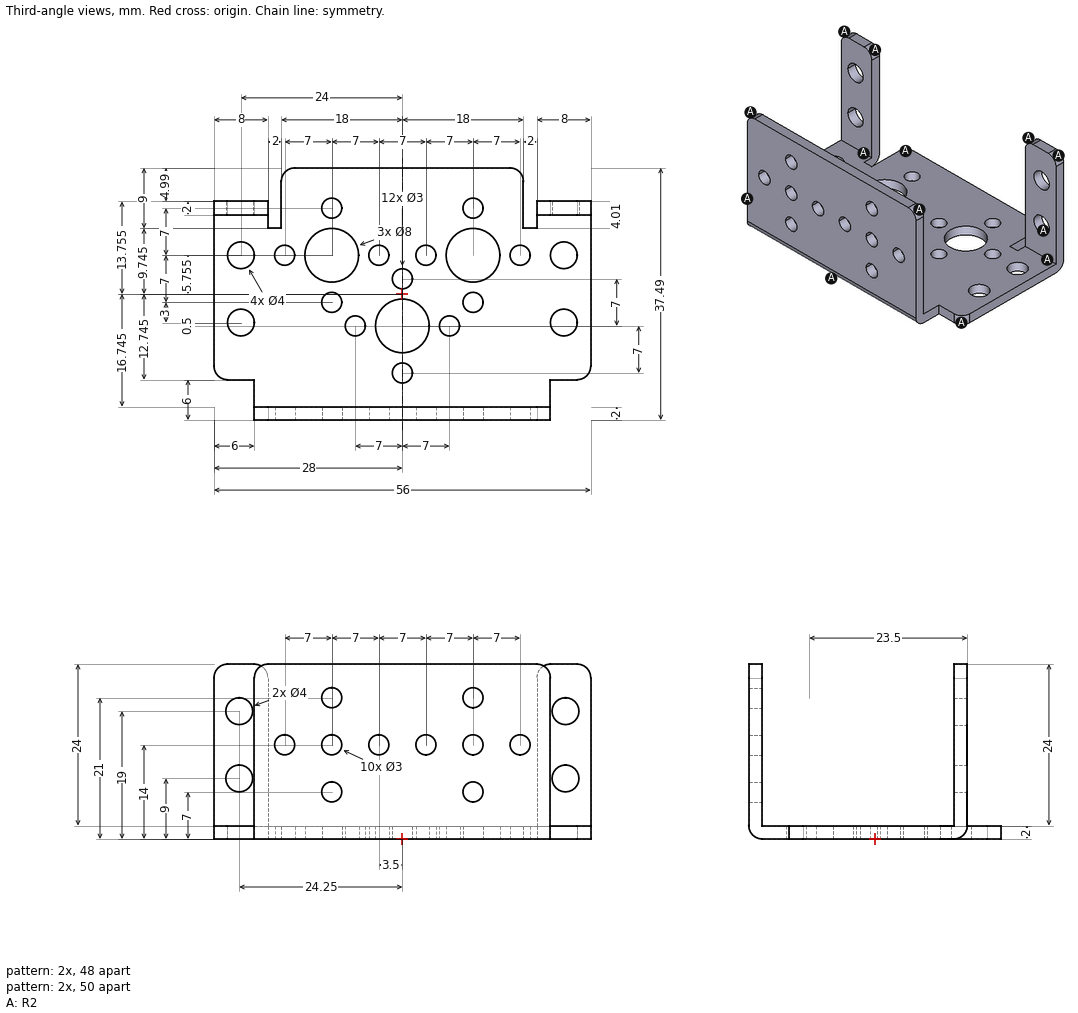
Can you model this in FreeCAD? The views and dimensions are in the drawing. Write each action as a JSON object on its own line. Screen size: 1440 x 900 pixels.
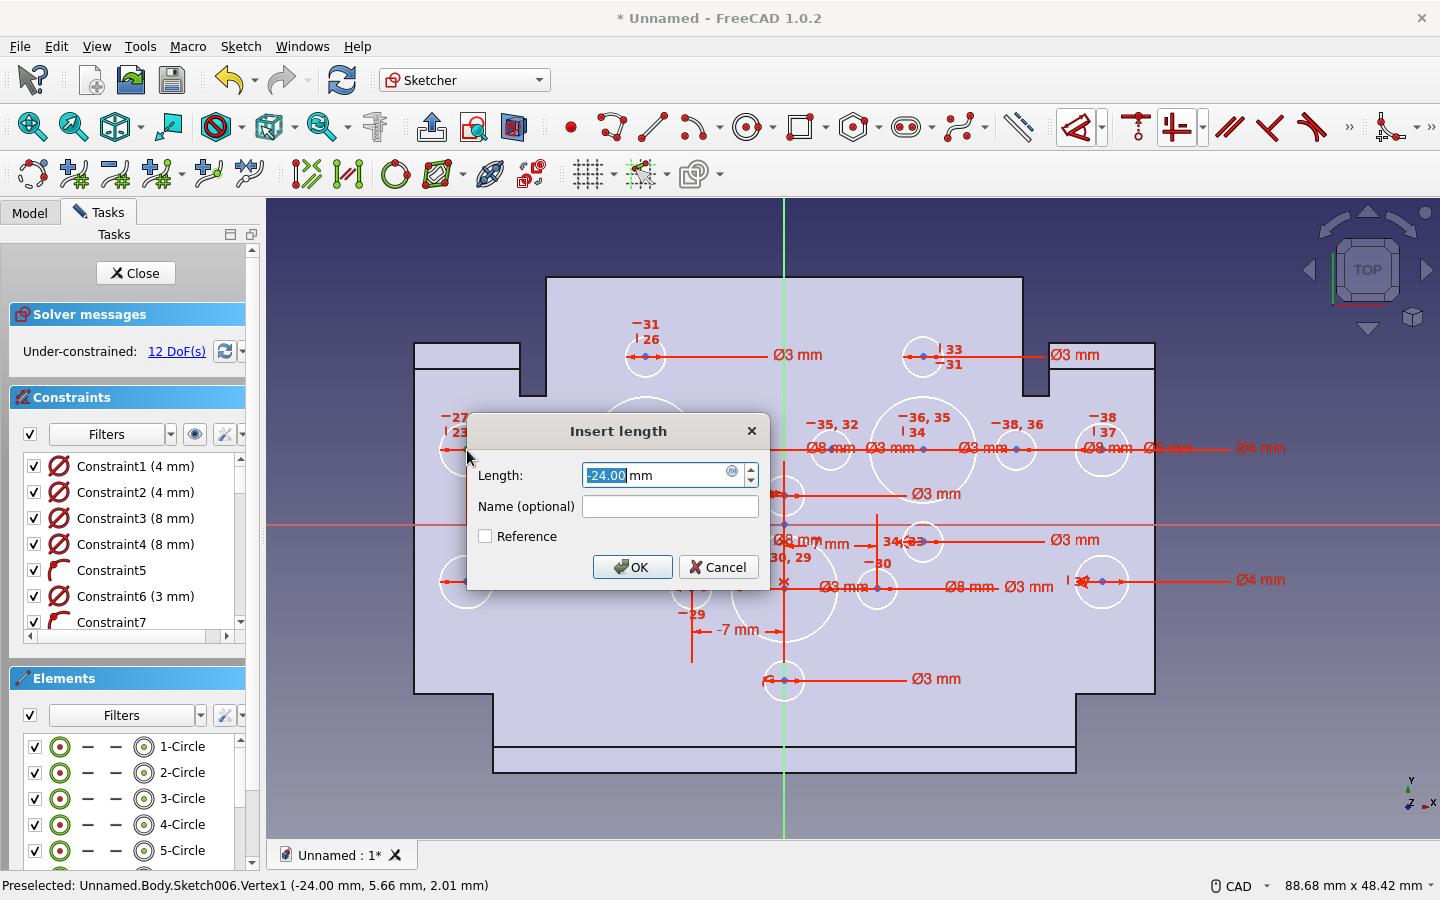
{"action": "type", "text": "-24"}
{"action": "key", "text": "Return"}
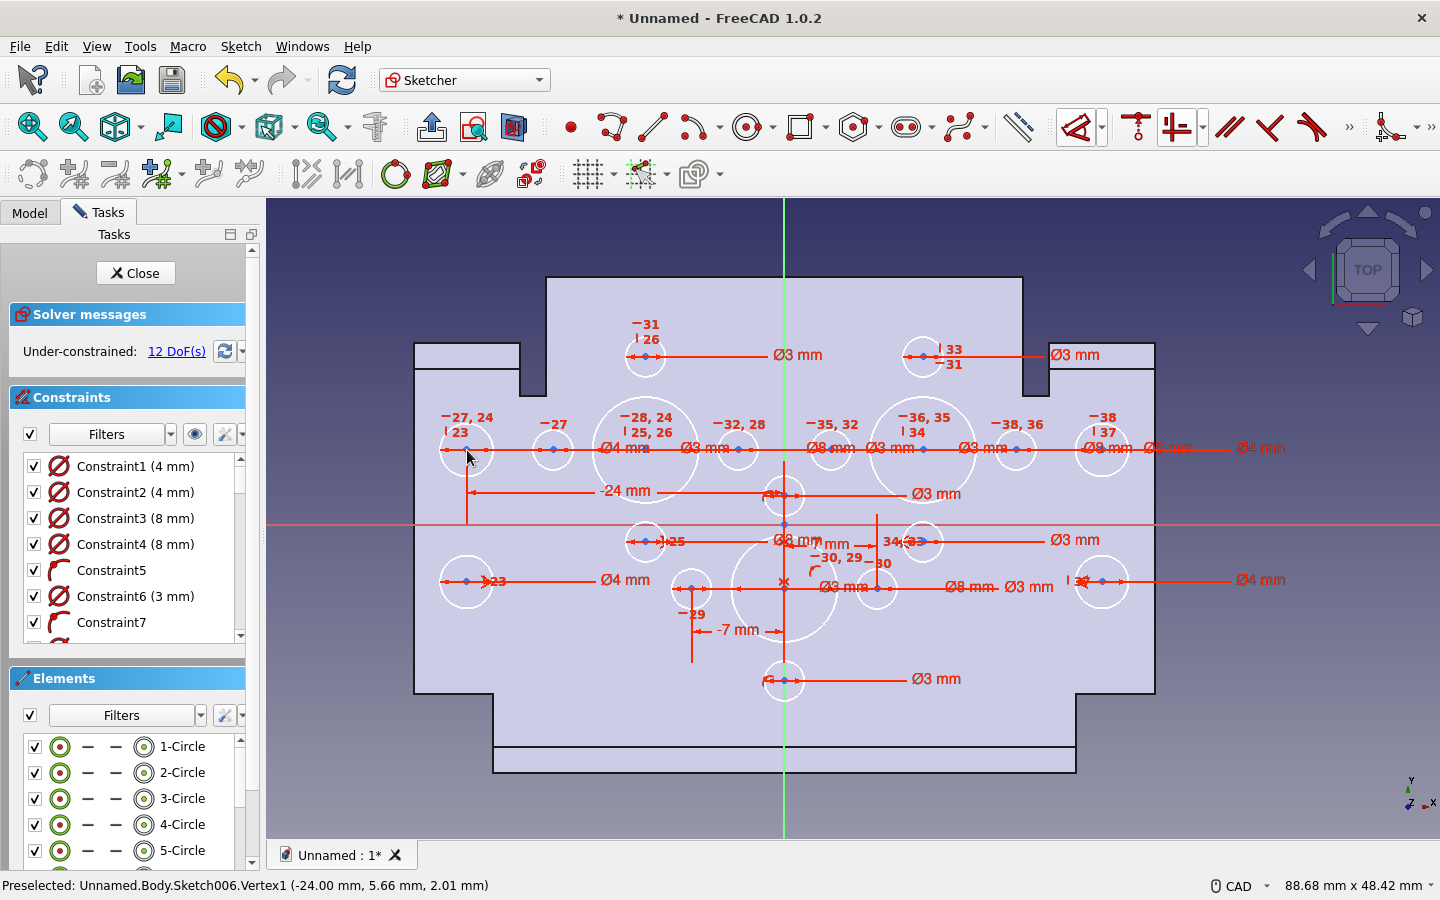
{"action": "left_click", "coordinate": [784, 589]}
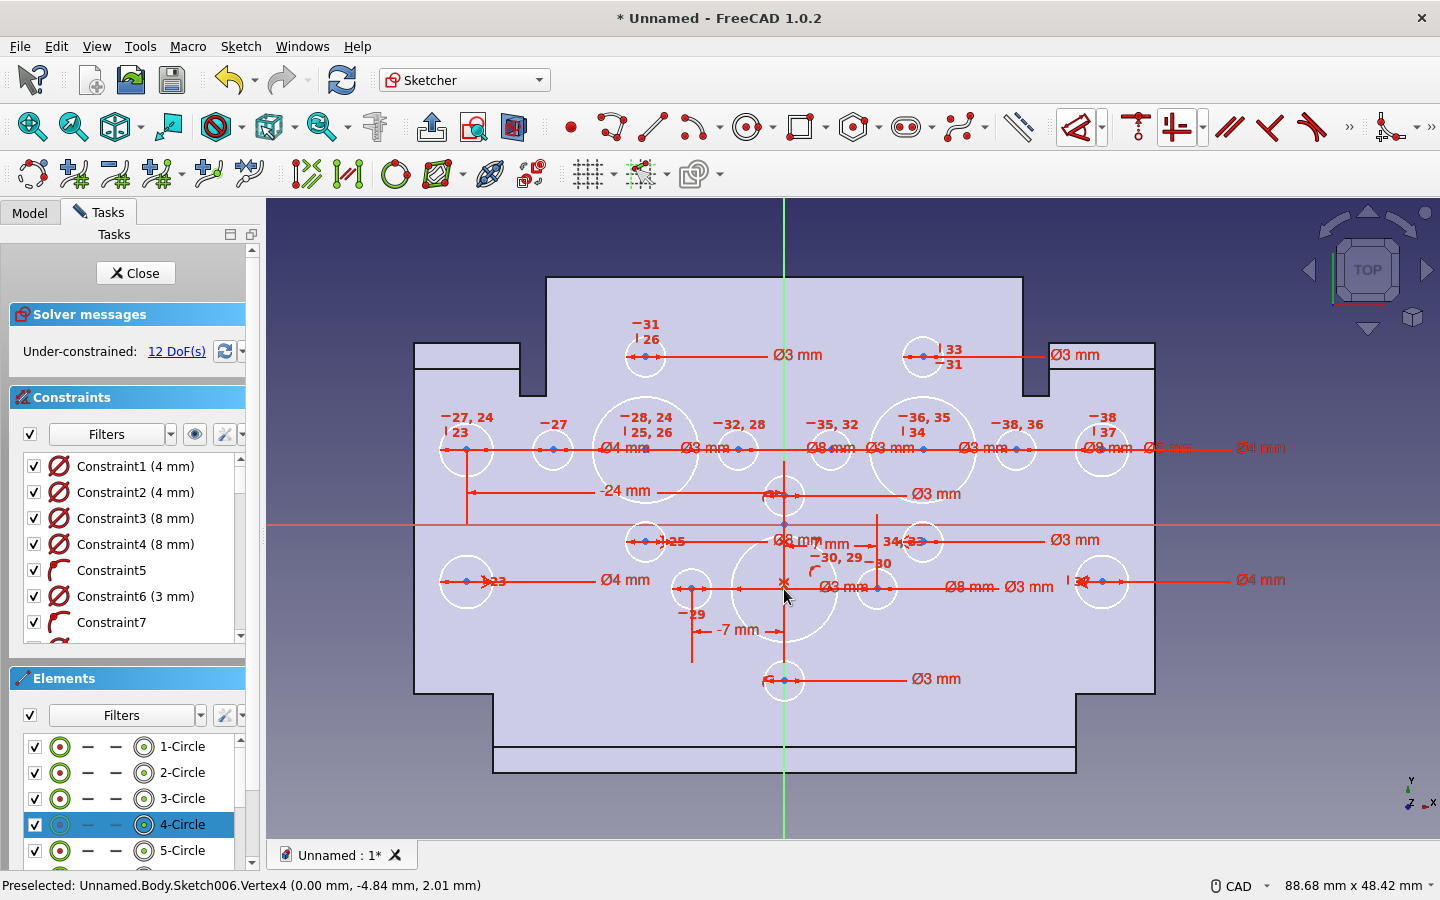
{"action": "left_click", "coordinate": [784, 496]}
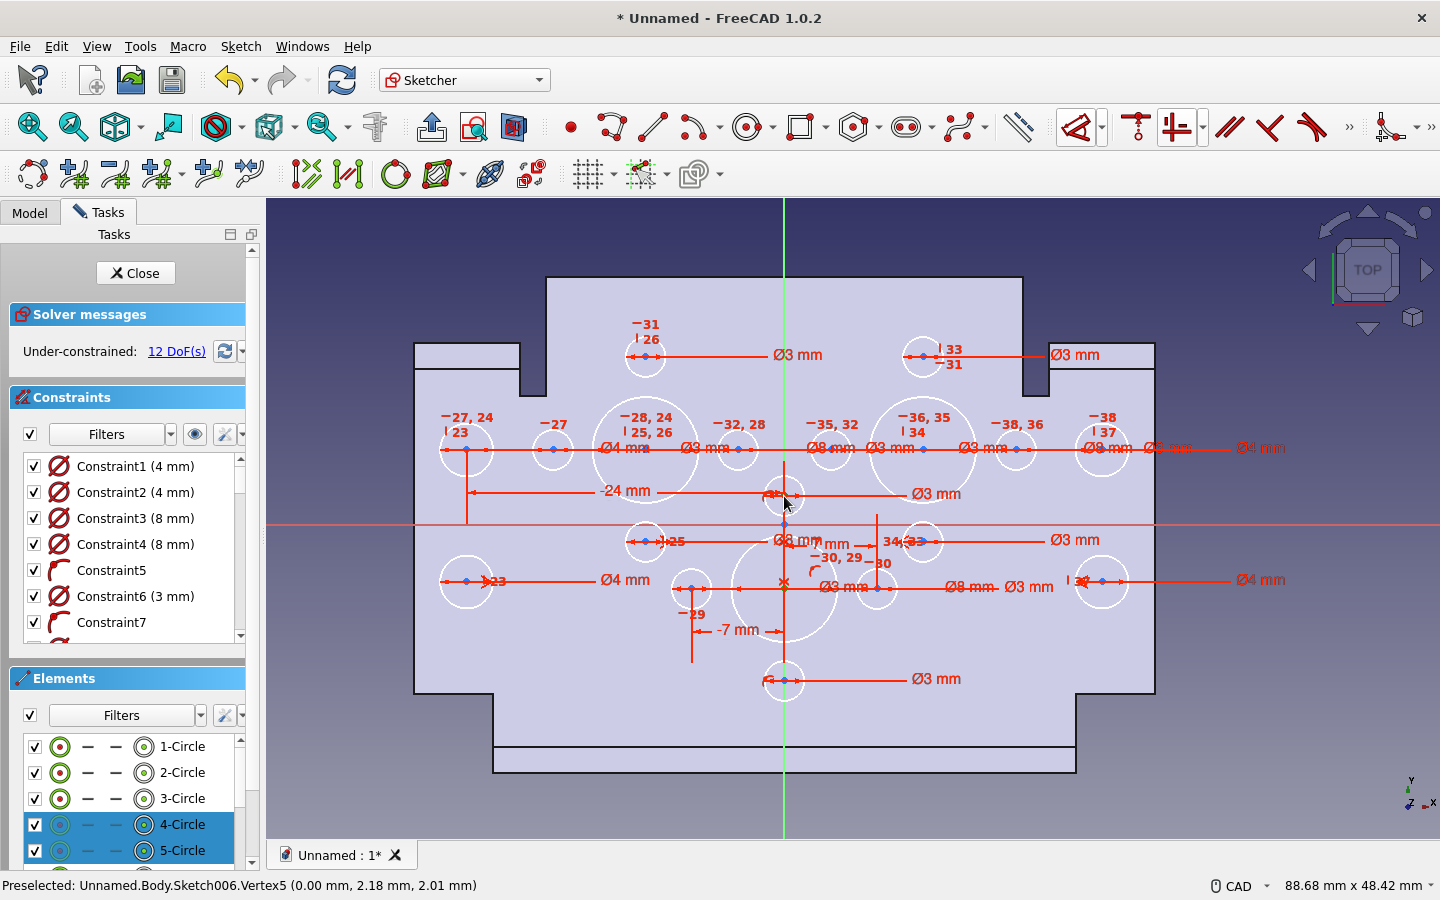
{"action": "key", "text": "i"}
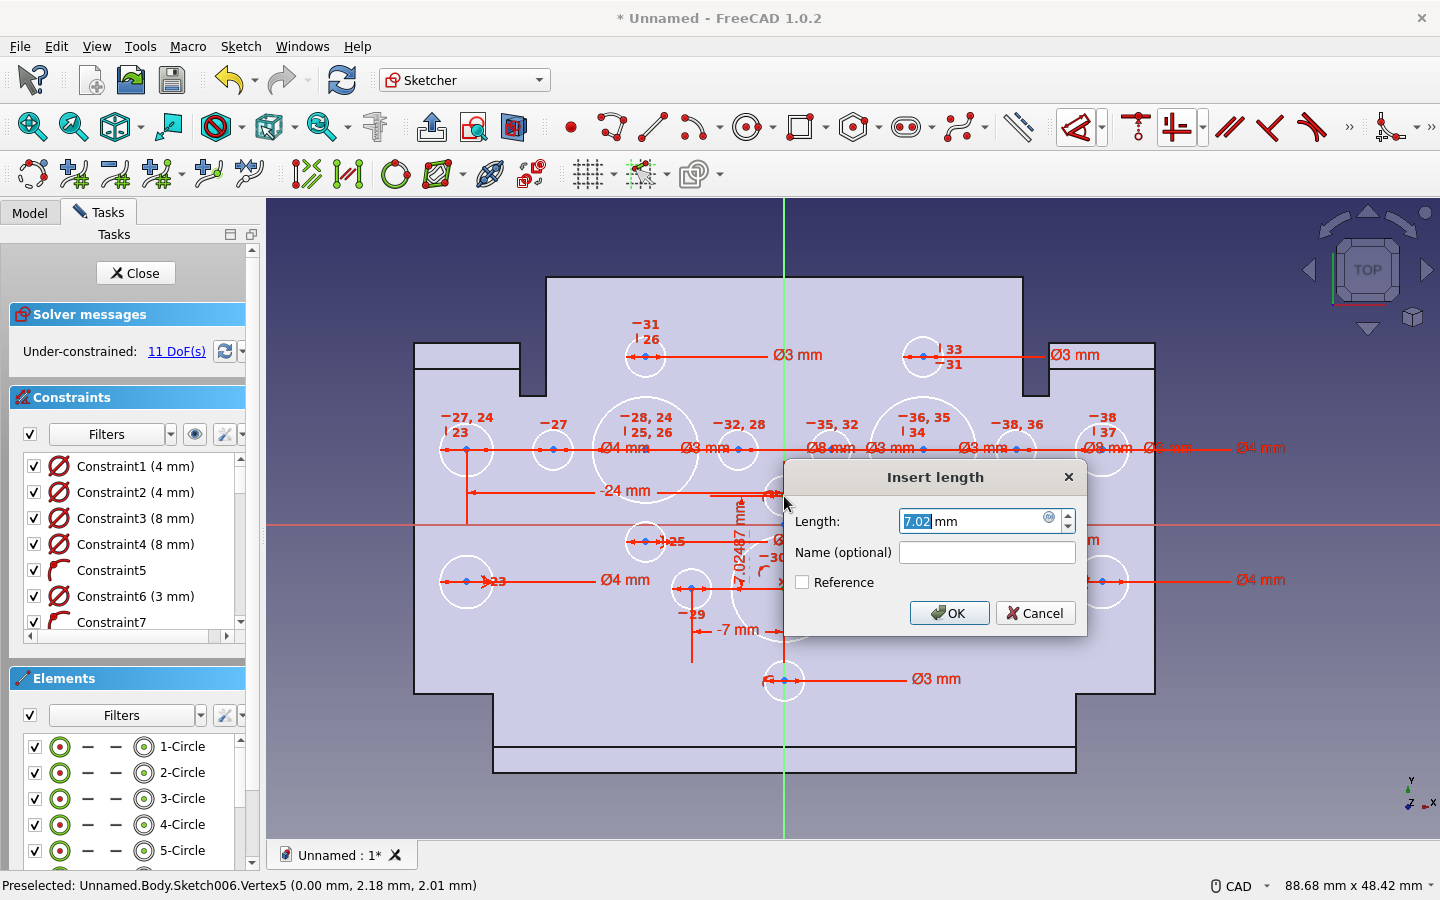
{"action": "type", "text": "7"}
{"action": "key", "text": "Return"}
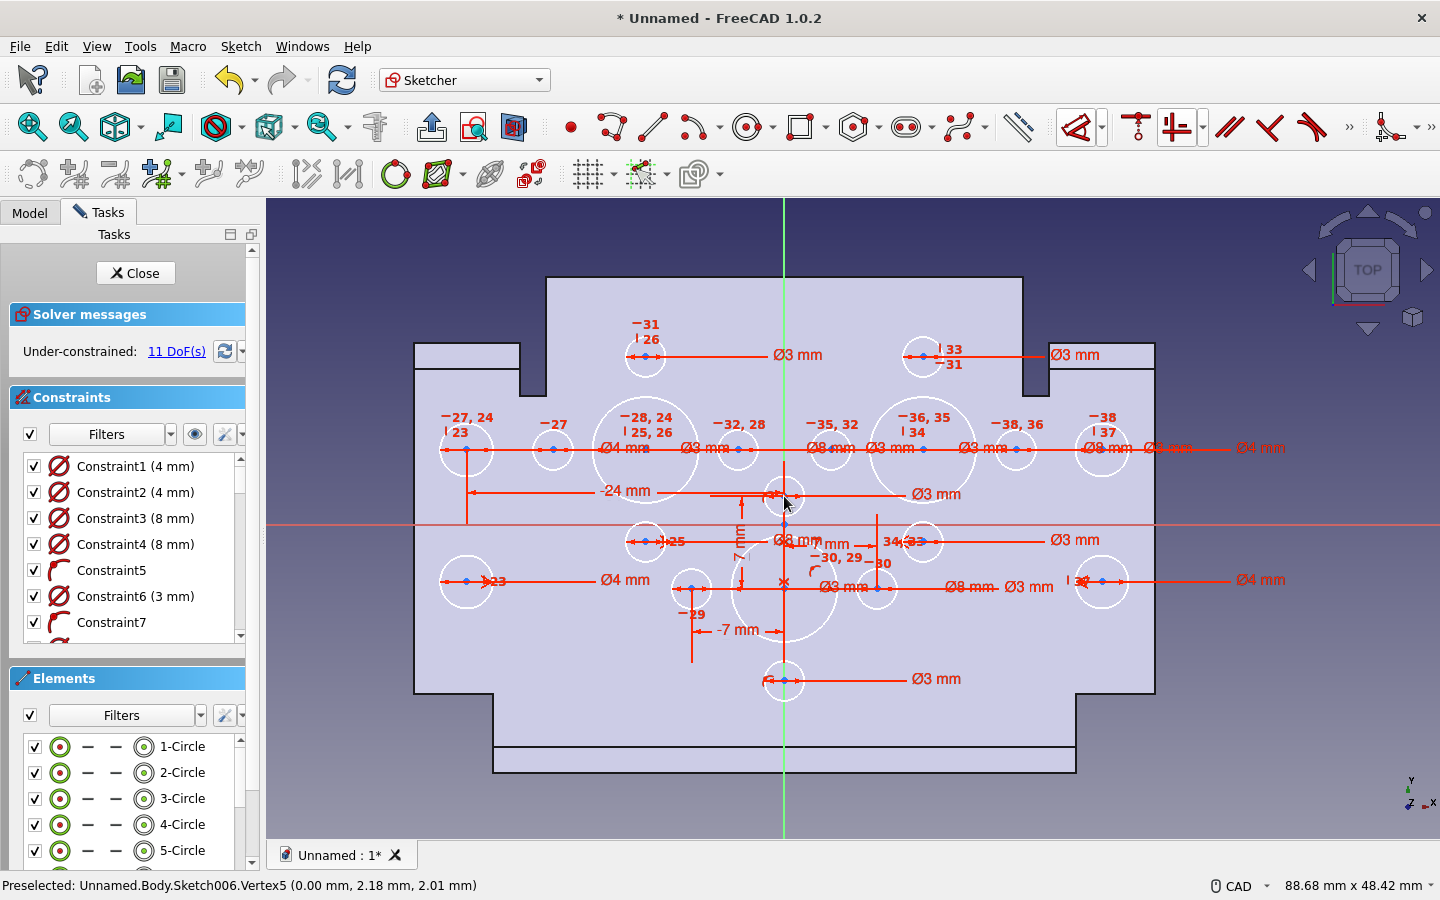
{"action": "left_click", "coordinate": [784, 589]}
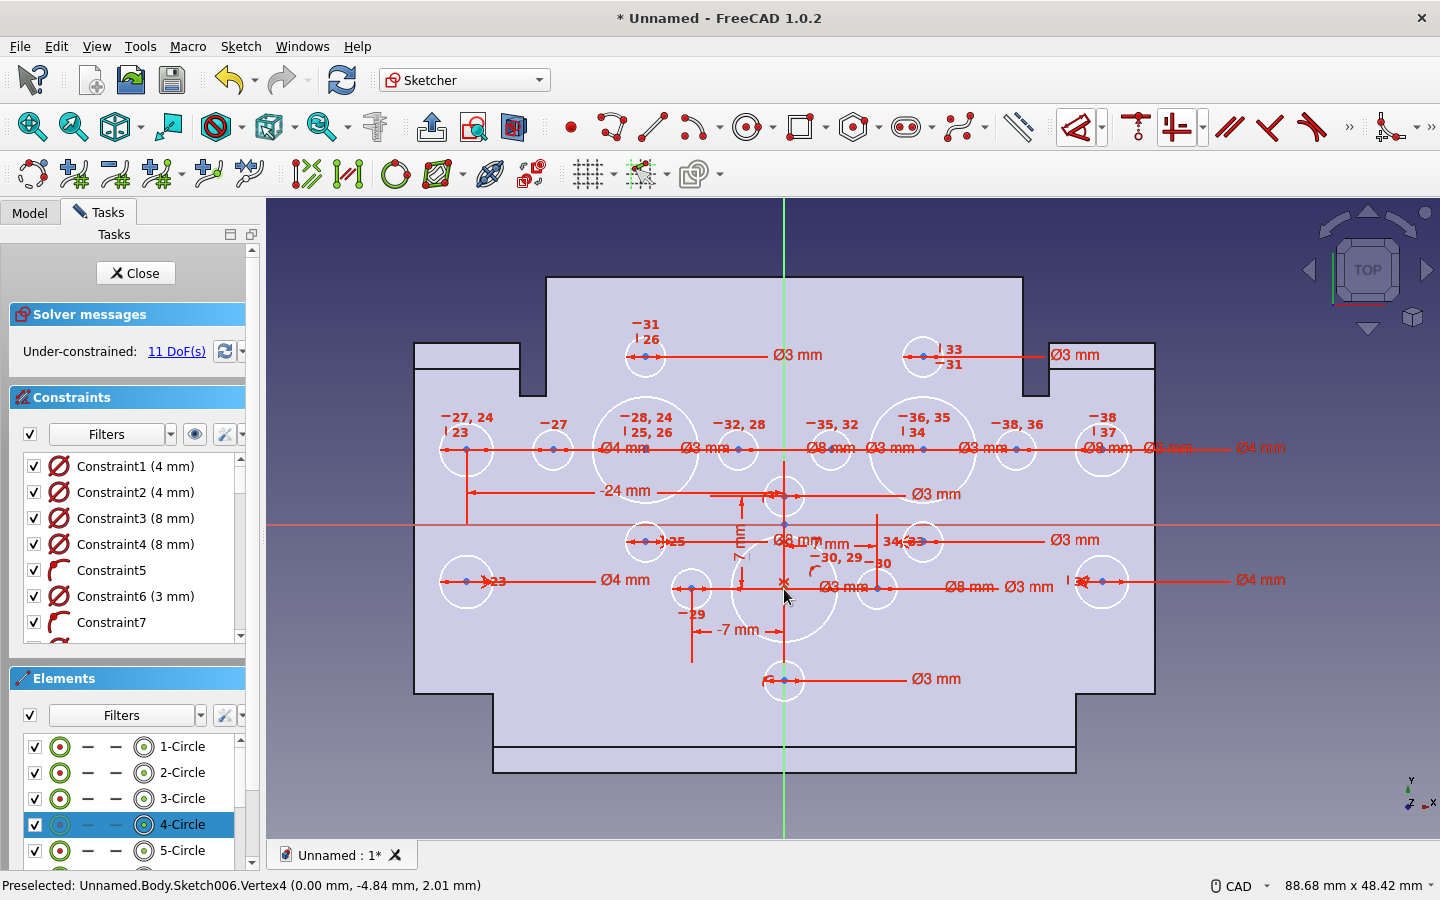
{"action": "left_click", "coordinate": [784, 681]}